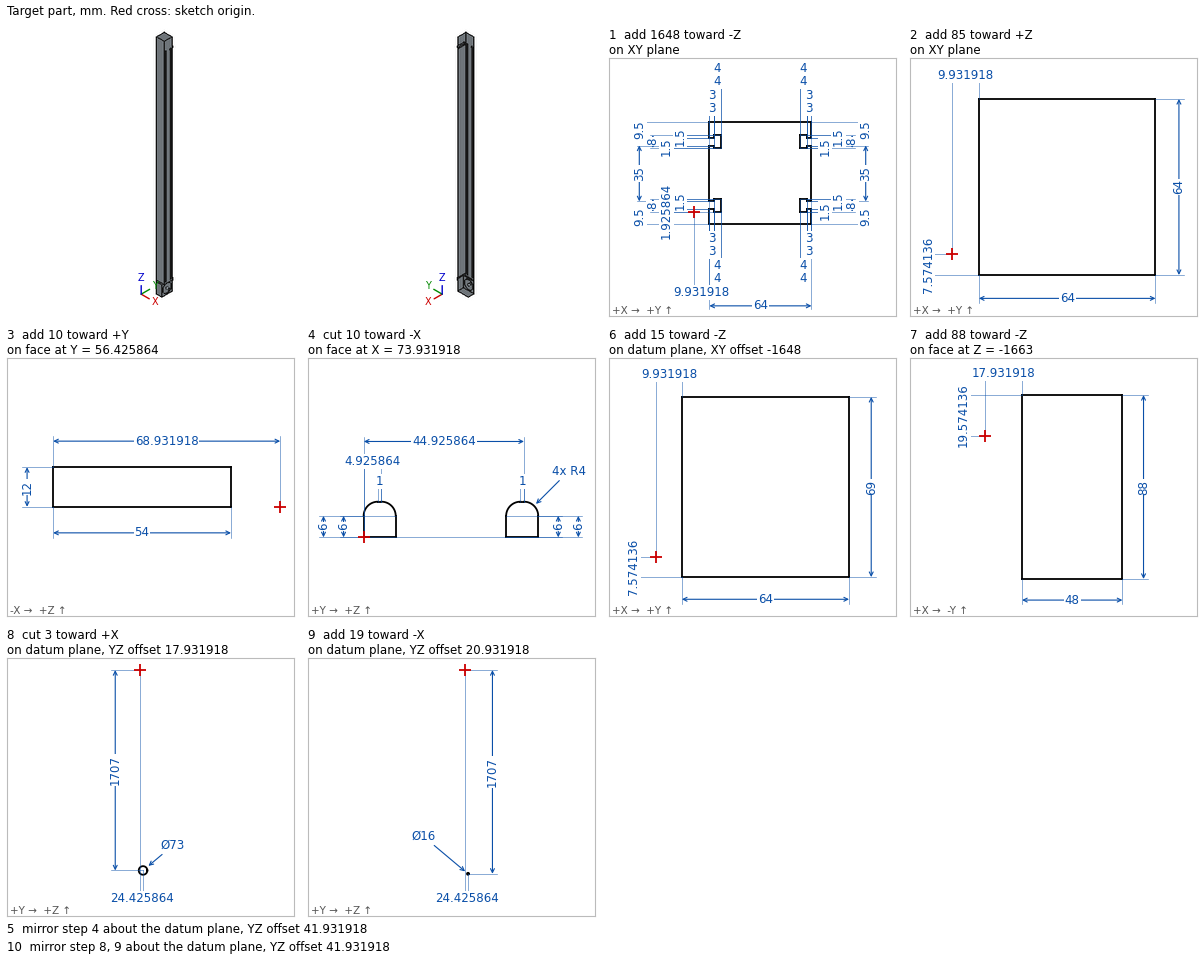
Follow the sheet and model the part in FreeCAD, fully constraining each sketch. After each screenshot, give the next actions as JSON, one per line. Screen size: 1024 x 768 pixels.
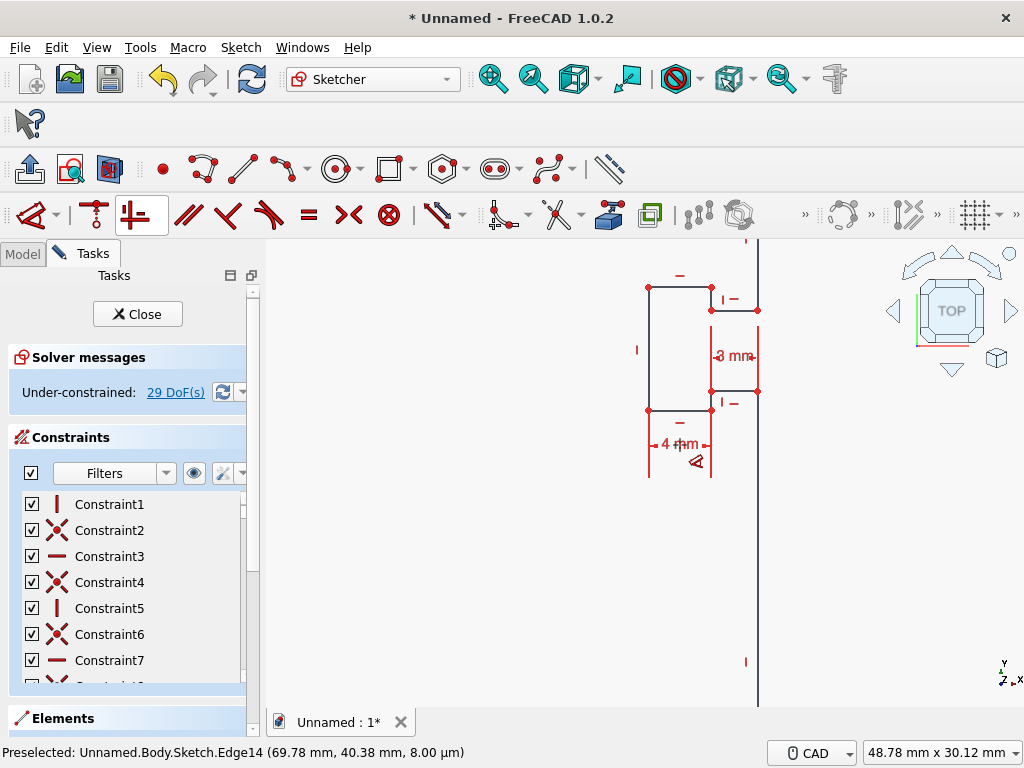
{"action": "left_click", "coordinate": [649, 374]}
{"action": "left_click", "coordinate": [683, 321]}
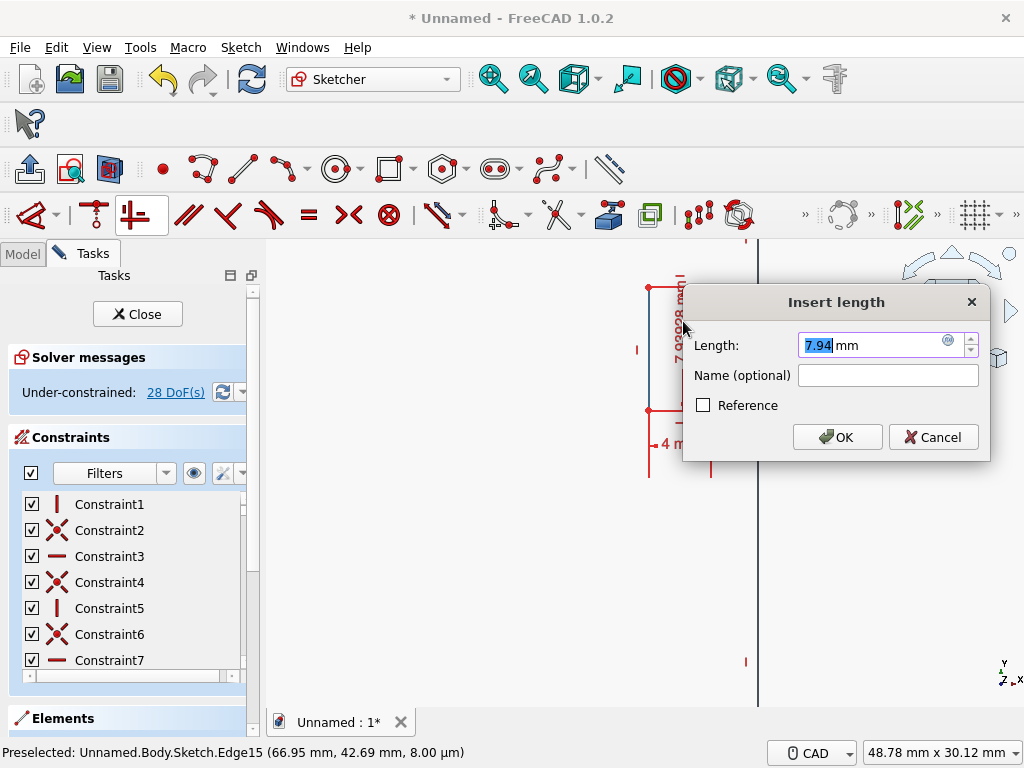
{"action": "type", "text": "8"}
{"action": "key", "text": "Return"}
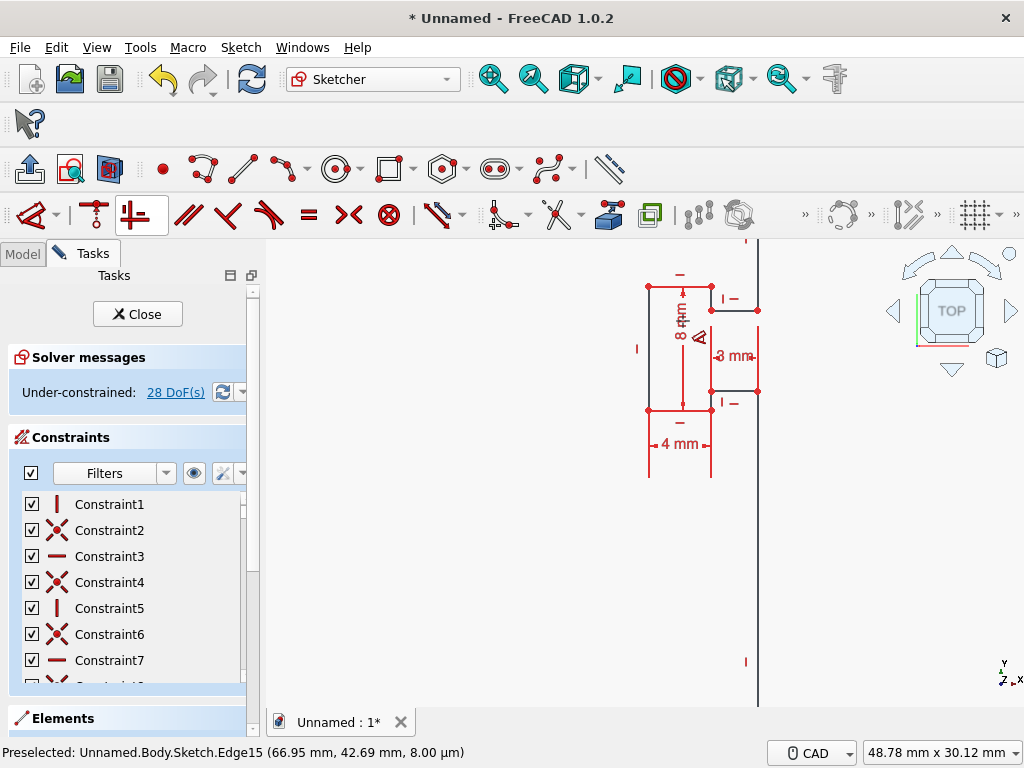
{"action": "left_click", "coordinate": [668, 287]}
{"action": "left_click", "coordinate": [680, 393]}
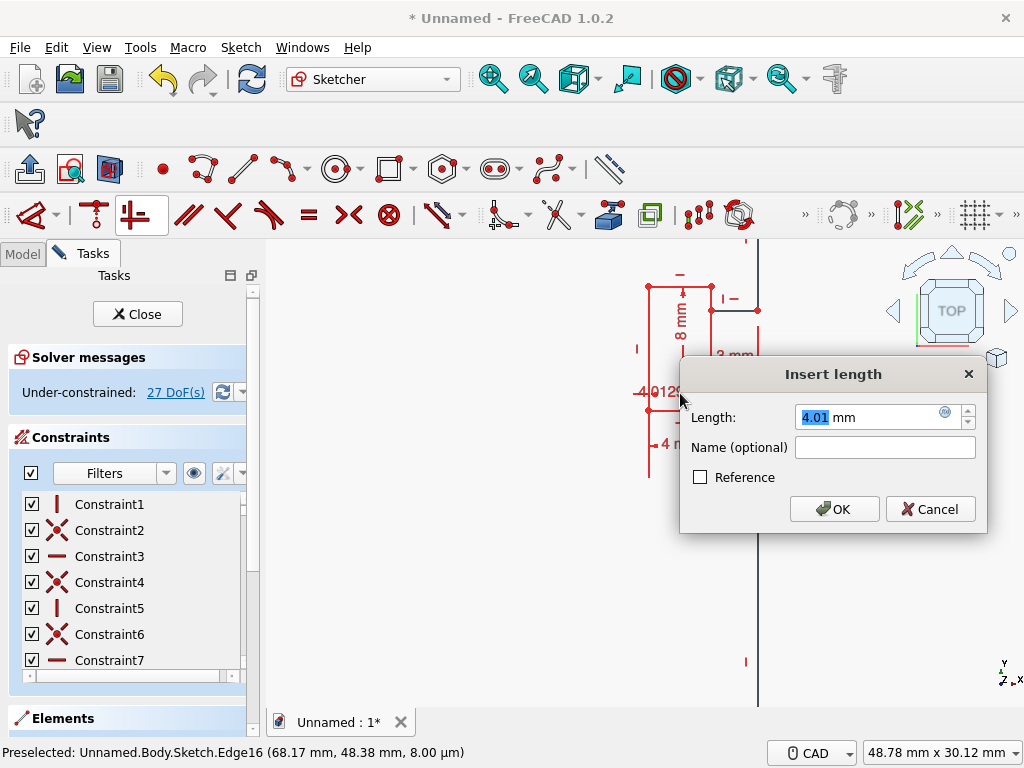
{"action": "type", "text": "4"}
{"action": "key", "text": "Return"}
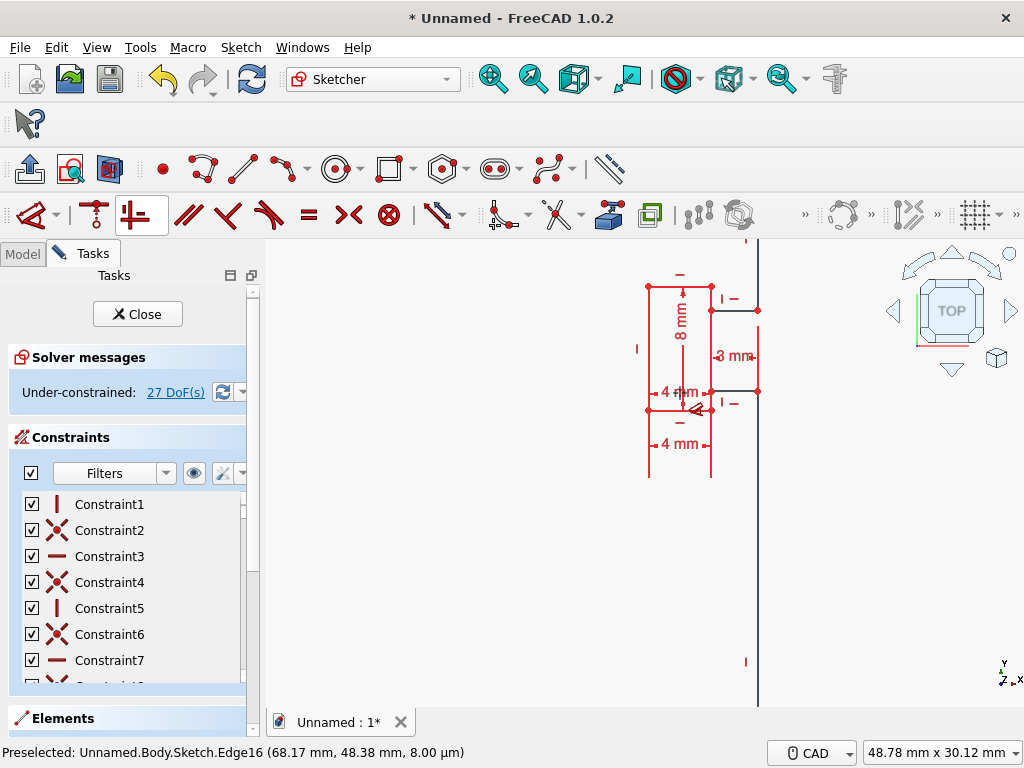
{"action": "left_click", "coordinate": [725, 311]}
{"action": "left_click", "coordinate": [734, 277]}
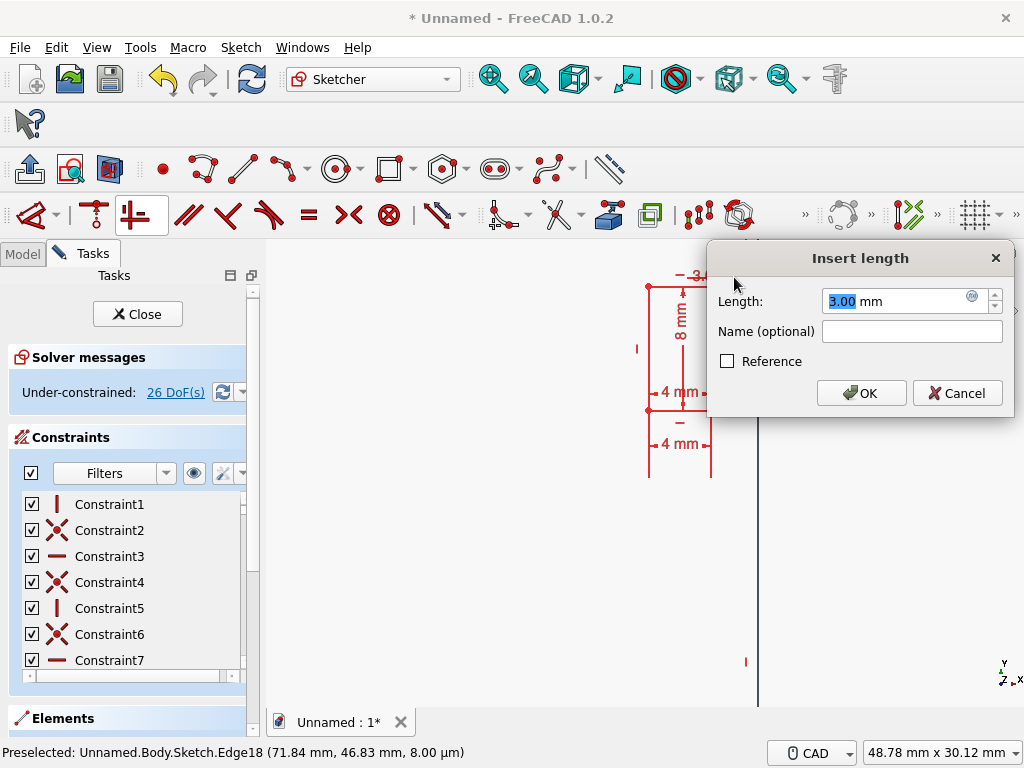
{"action": "type", "text": "3"}
{"action": "key", "text": "Return"}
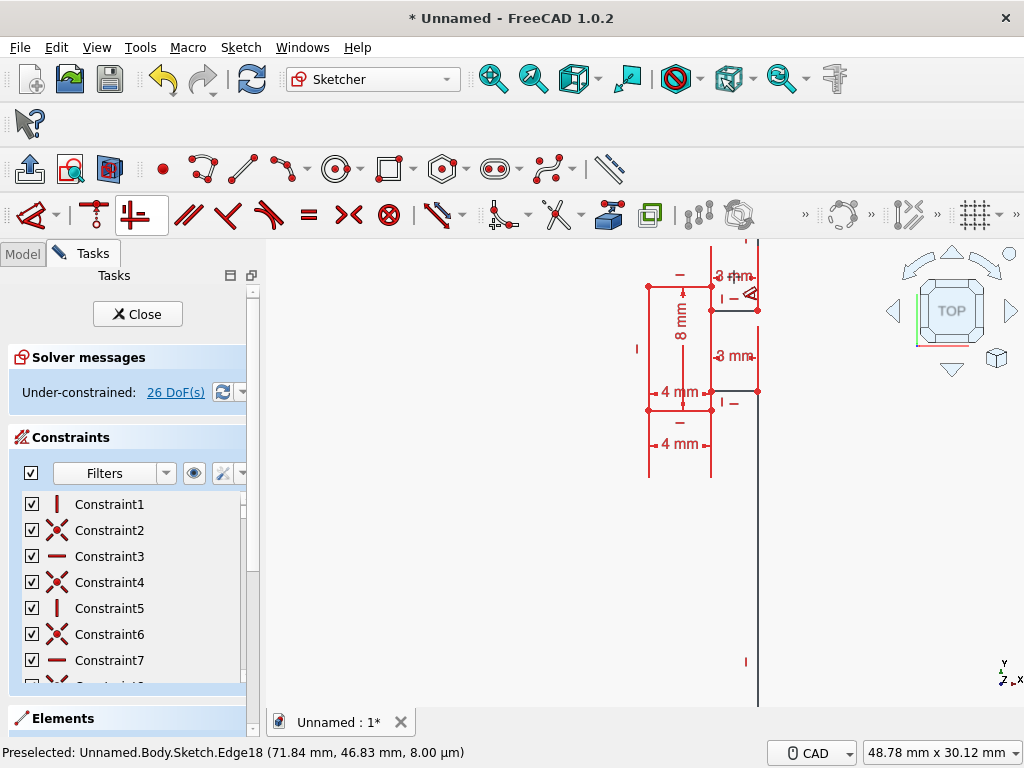
{"action": "scroll", "coordinate": [746, 393], "scroll_direction": "down", "scroll_amount": 6}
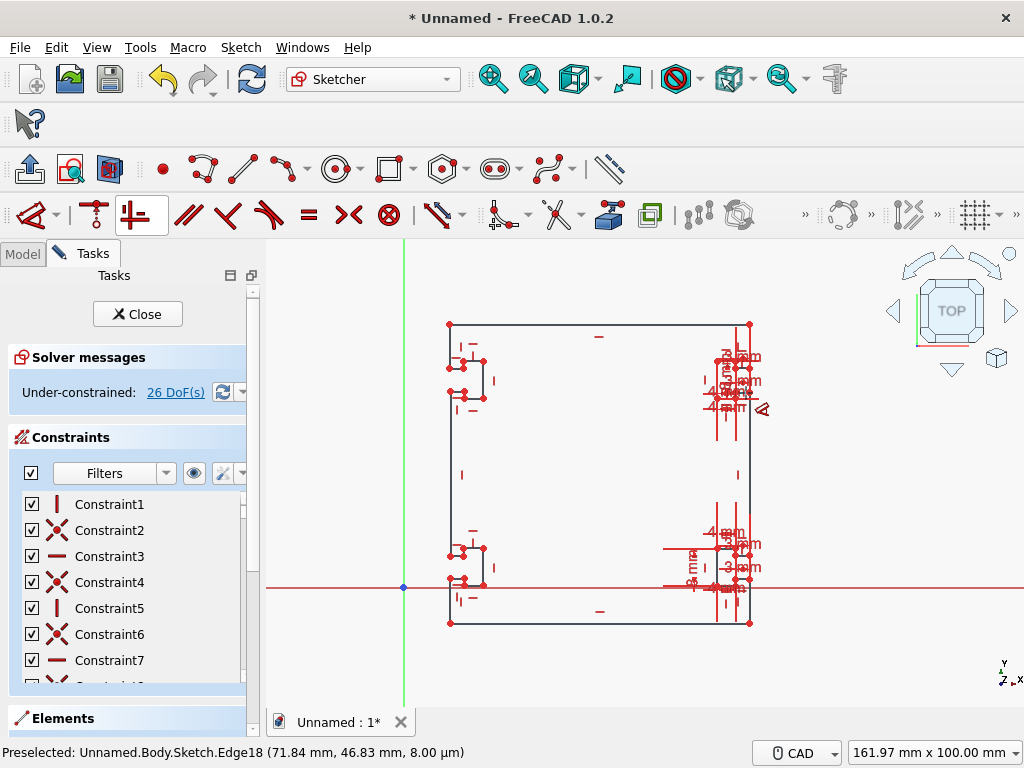
{"action": "scroll", "coordinate": [454, 369], "scroll_direction": "up", "scroll_amount": 6}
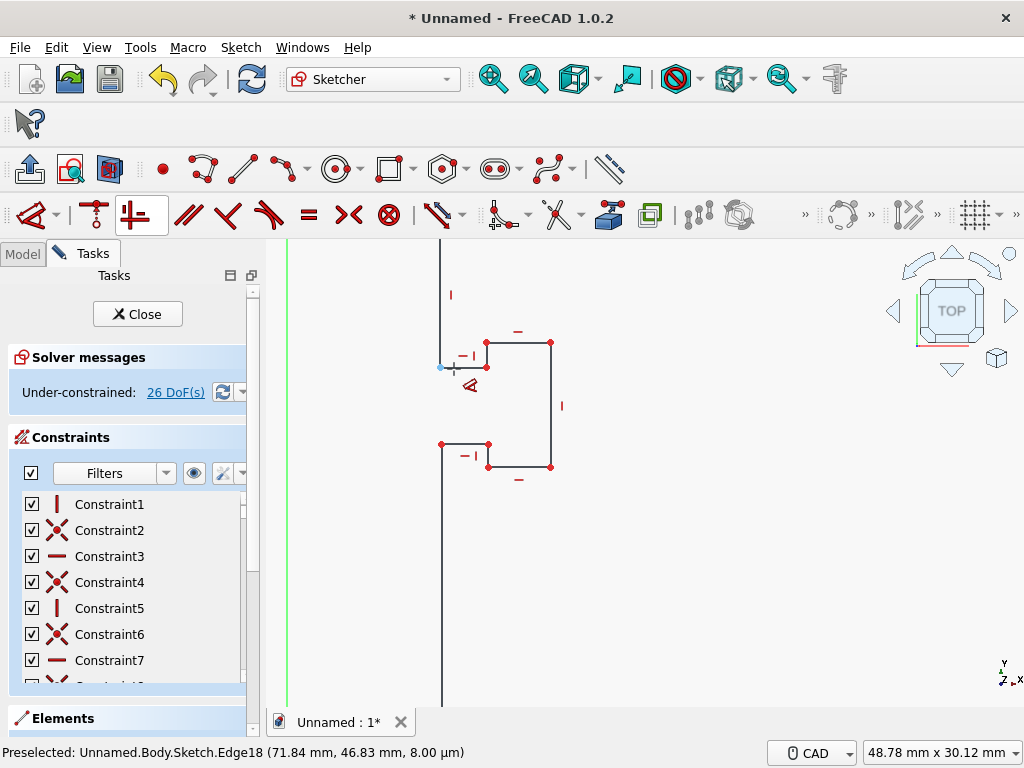
{"action": "left_click", "coordinate": [454, 368]}
{"action": "left_click", "coordinate": [463, 334]}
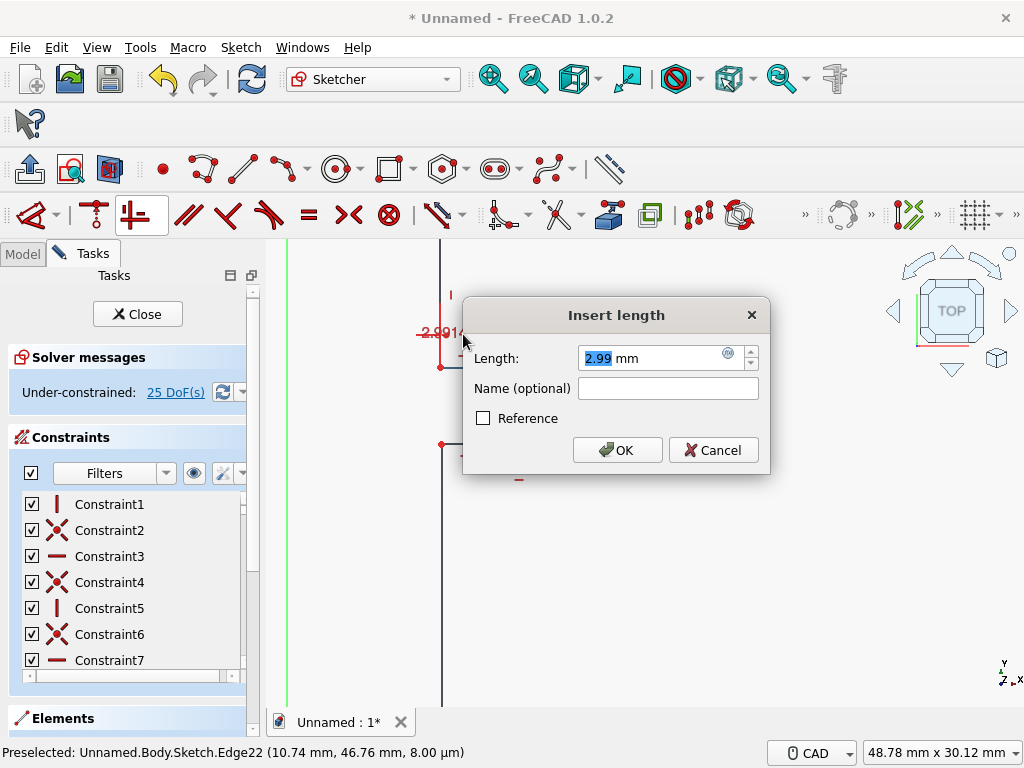
{"action": "type", "text": "3"}
{"action": "key", "text": "Return"}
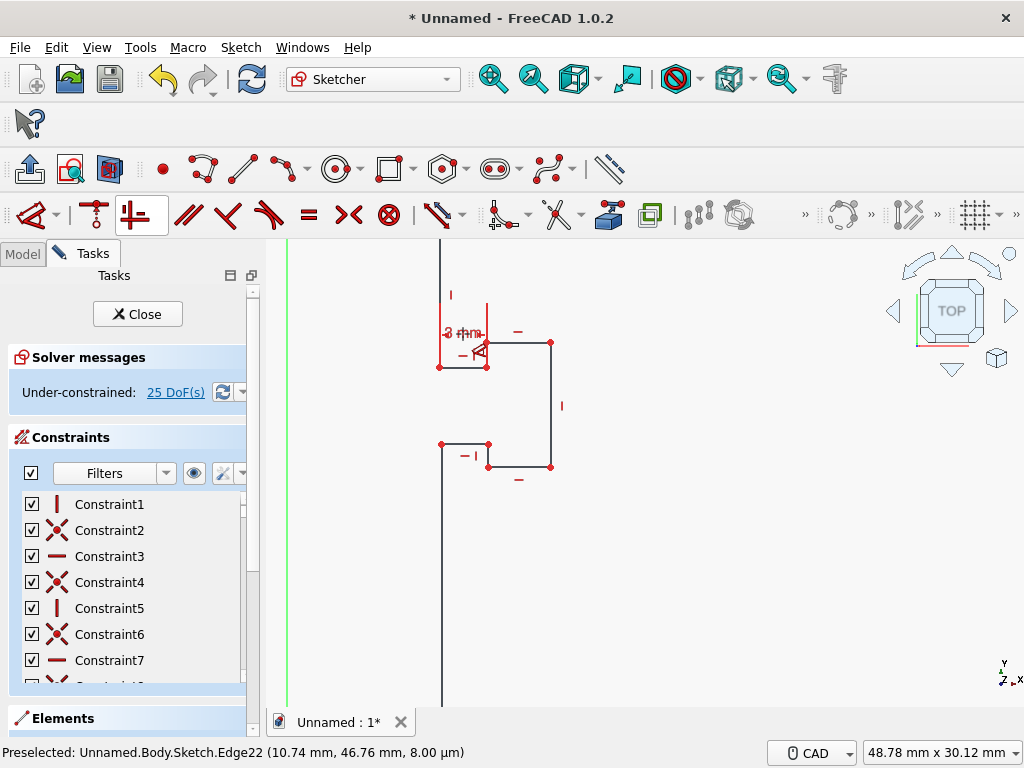
{"action": "left_click", "coordinate": [506, 343]}
{"action": "left_click", "coordinate": [519, 309]}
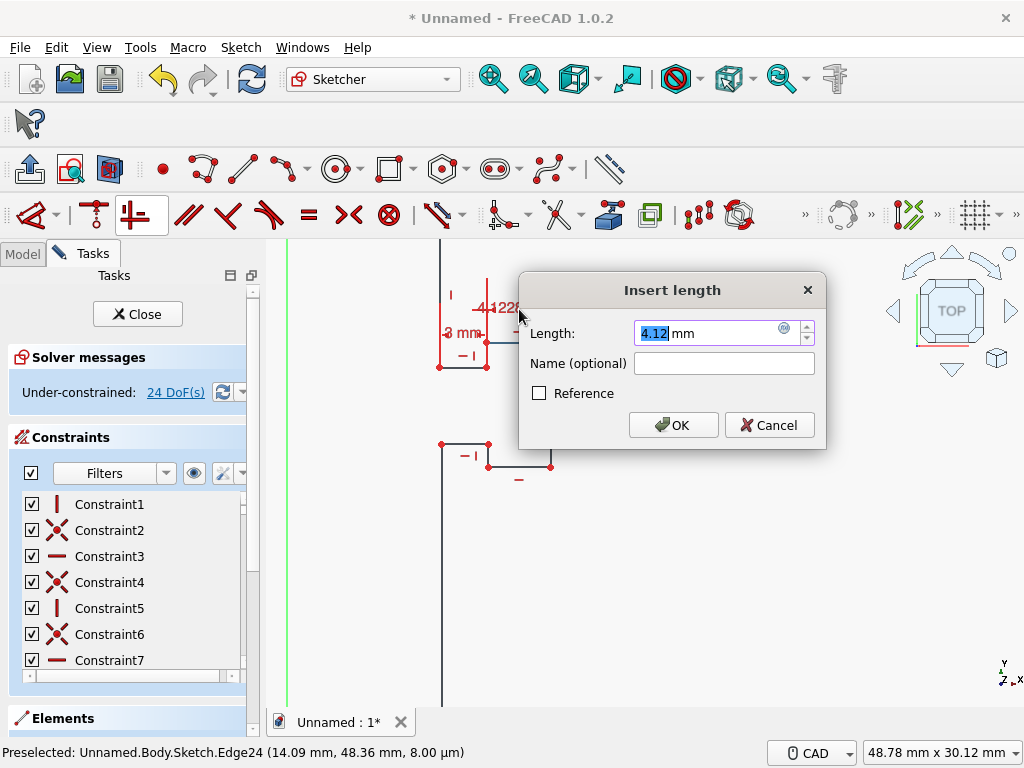
{"action": "type", "text": "4"}
{"action": "key", "text": "Return"}